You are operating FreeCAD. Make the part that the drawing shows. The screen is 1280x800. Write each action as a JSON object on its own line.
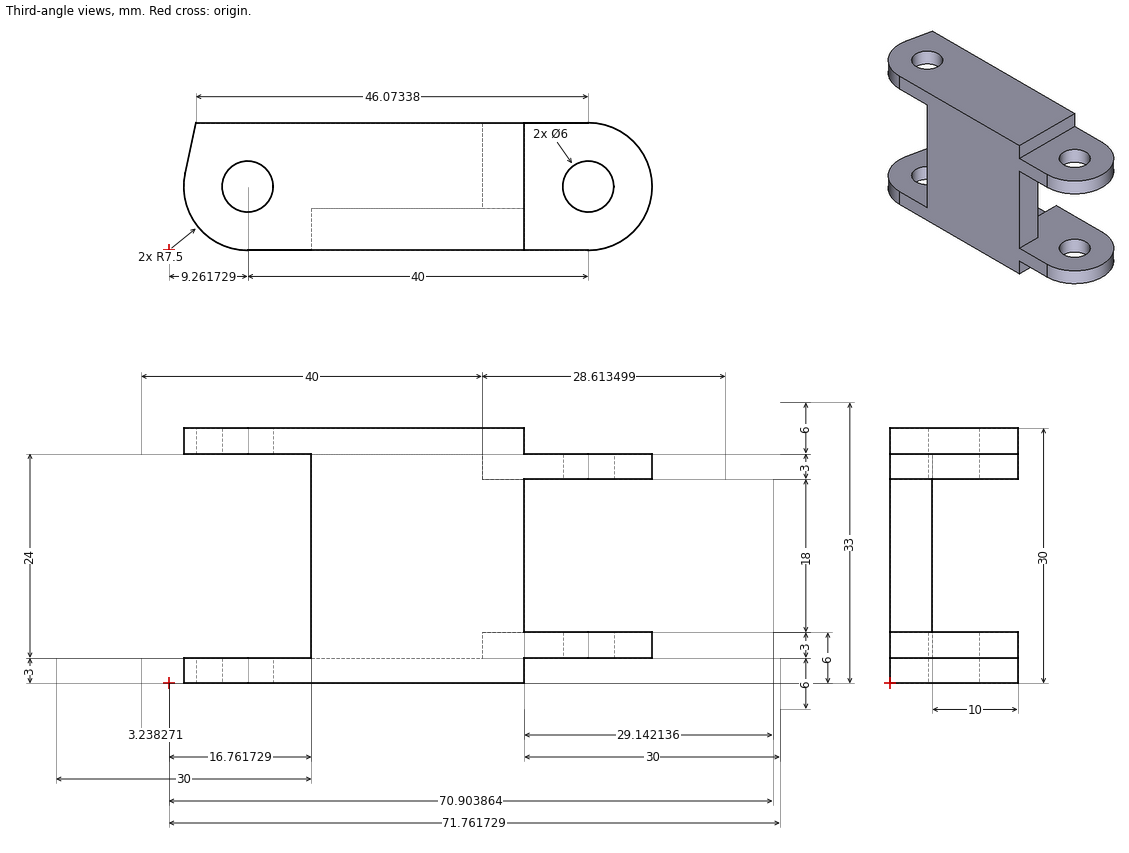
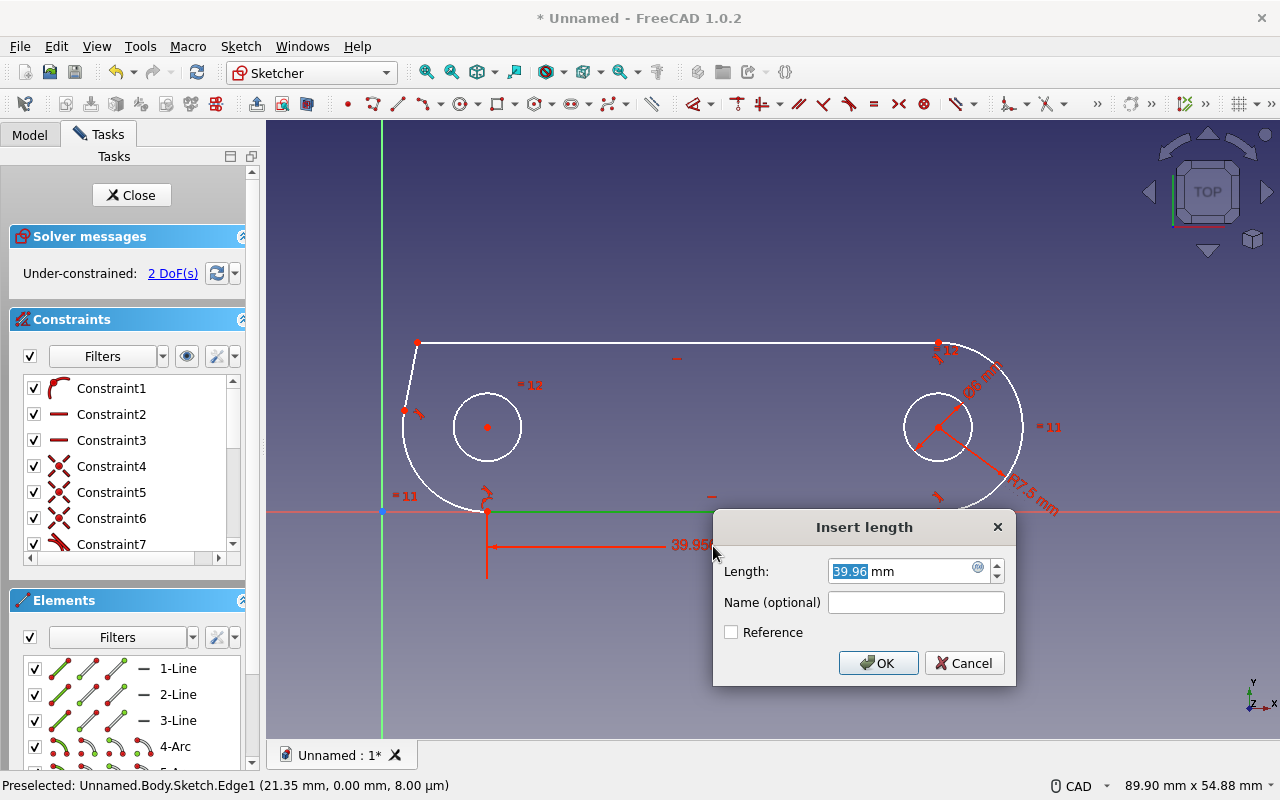
{"action": "type", "text": "40"}
{"action": "key", "text": "Return"}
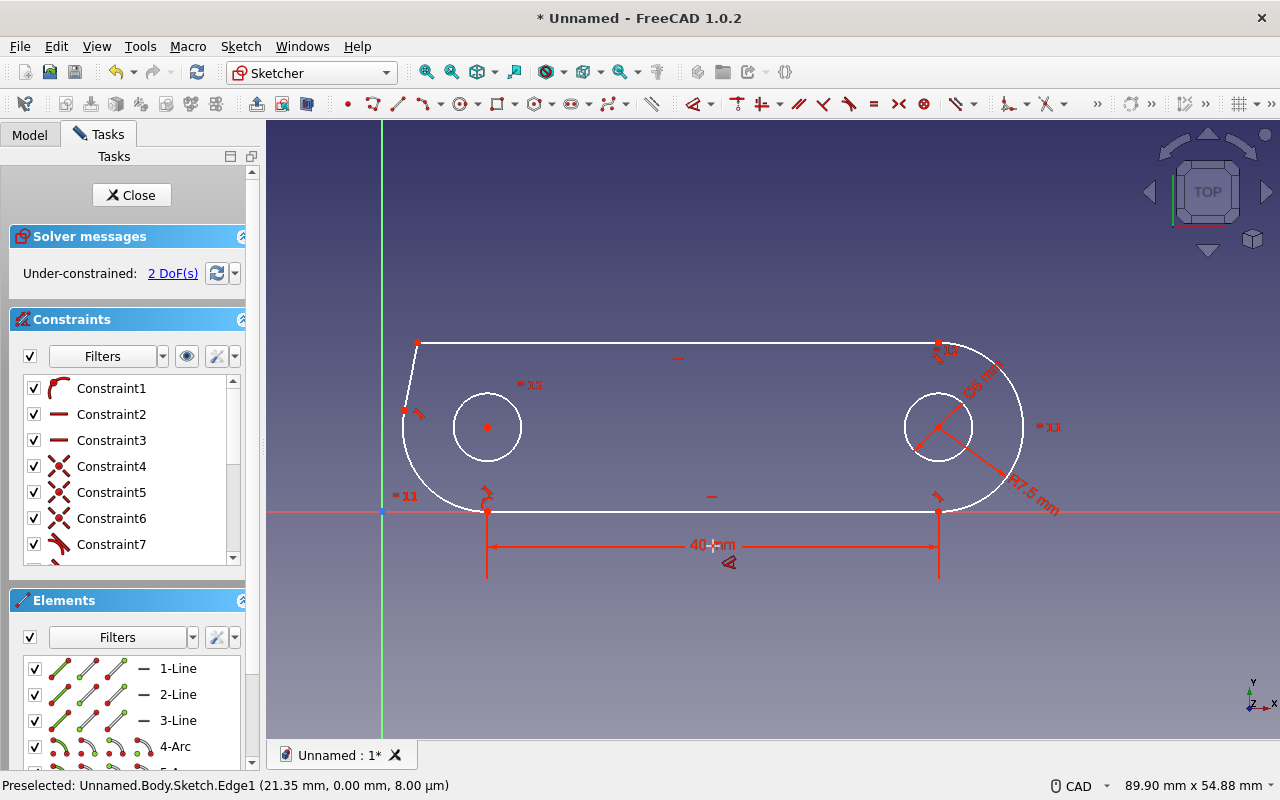
{"action": "left_click", "coordinate": [782, 343]}
{"action": "left_click", "coordinate": [678, 309]}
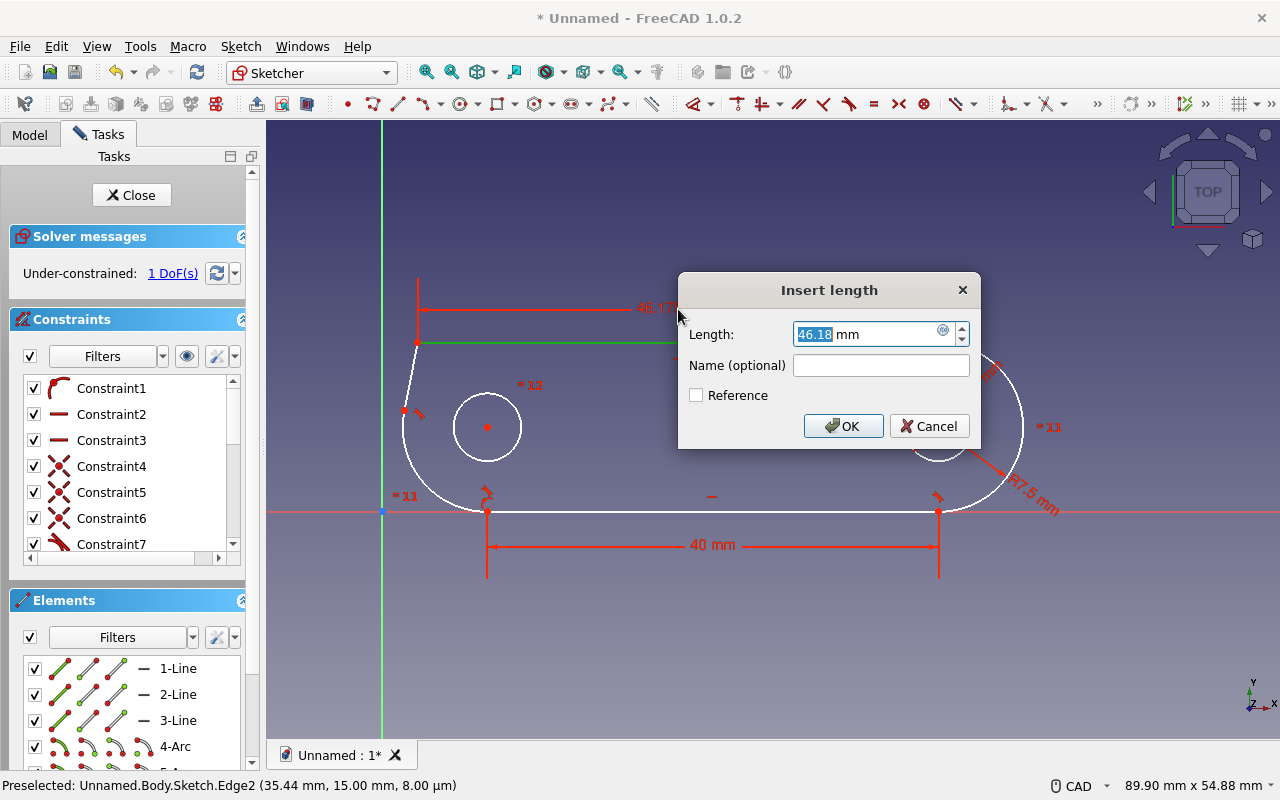
{"action": "type", "text": "46.07338"}
{"action": "key", "text": "Return"}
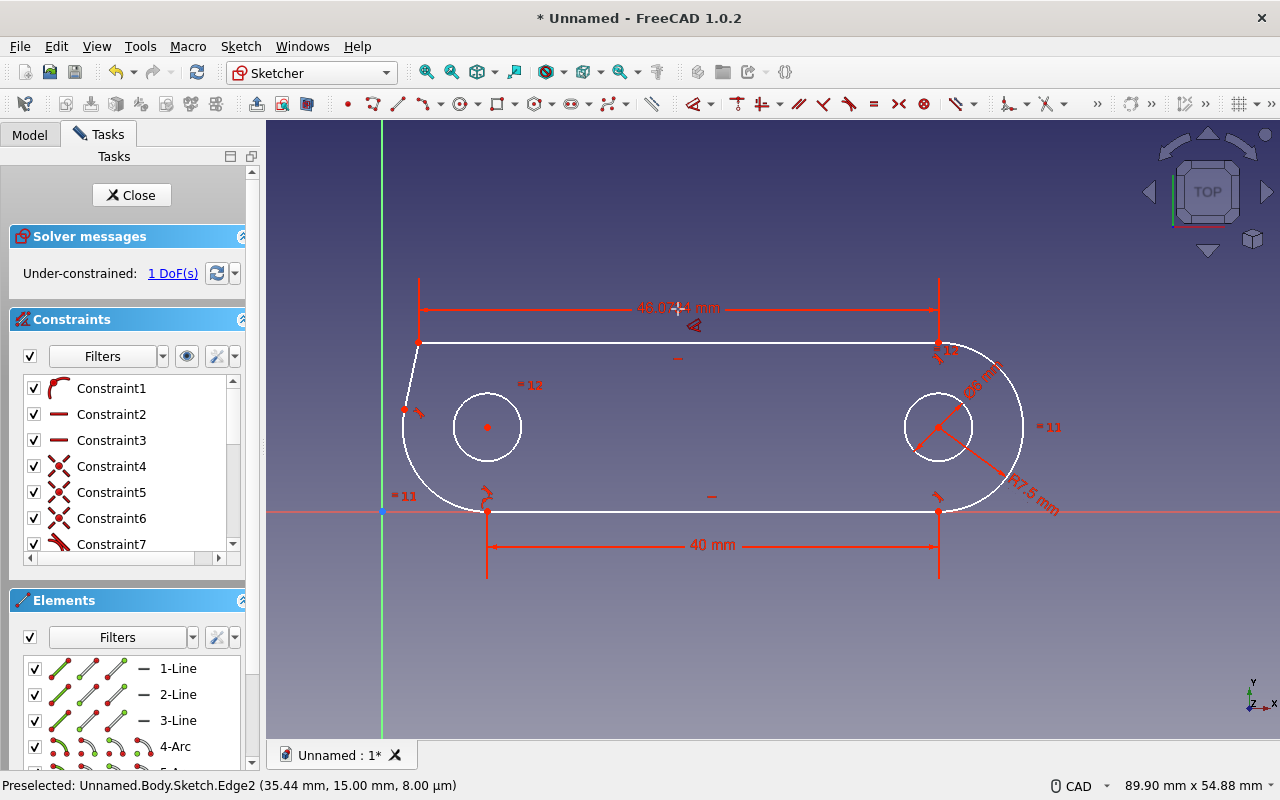
{"action": "left_click", "coordinate": [487, 427]}
{"action": "left_click", "coordinate": [435, 546]}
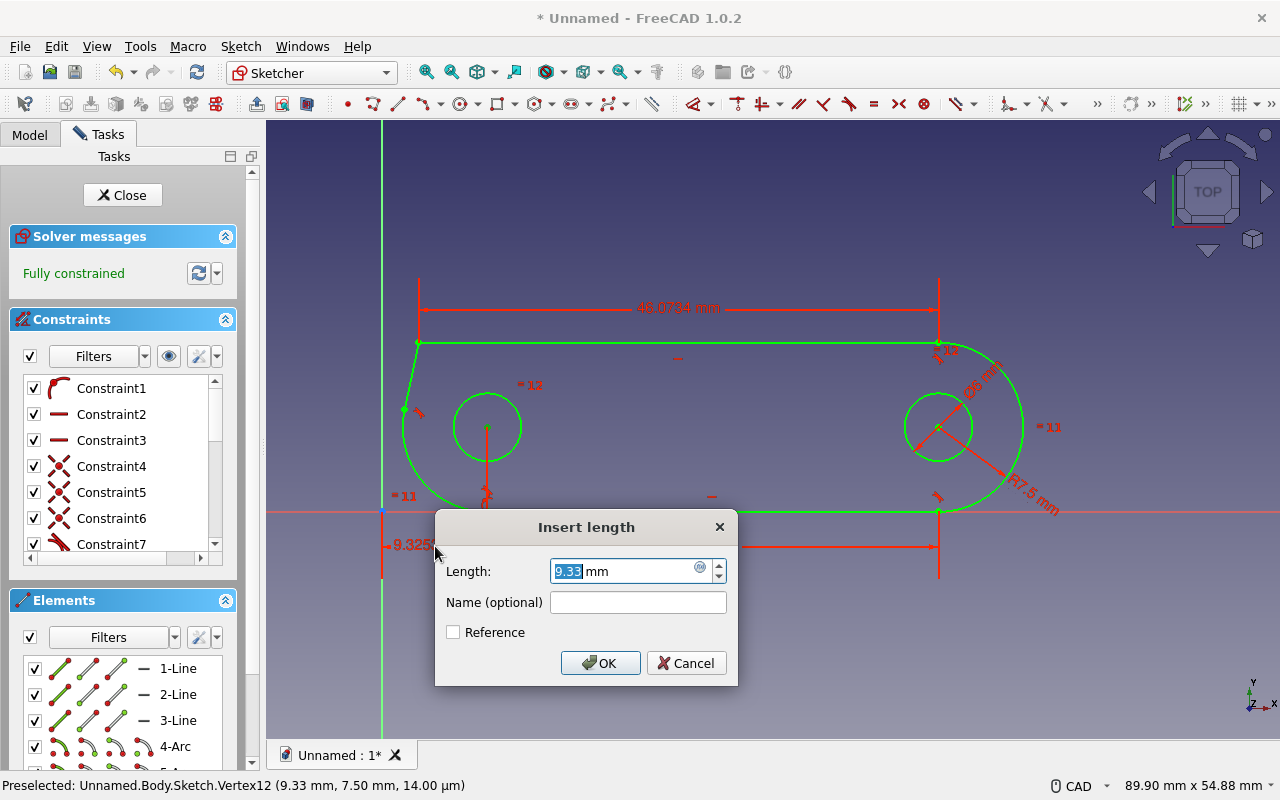
{"action": "type", "text": "9.261729"}
{"action": "key", "text": "Return"}
{"action": "key", "text": "Escape"}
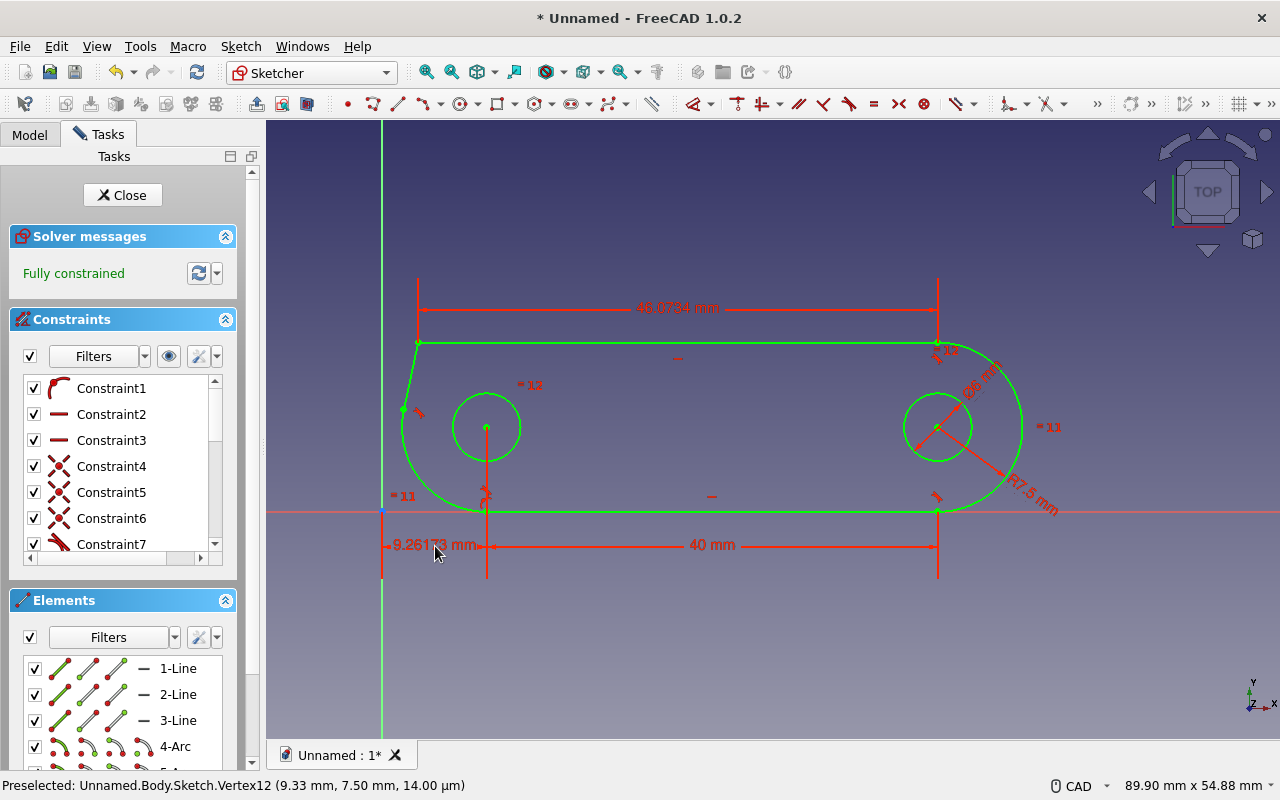
{"action": "left_click", "coordinate": [123, 195]}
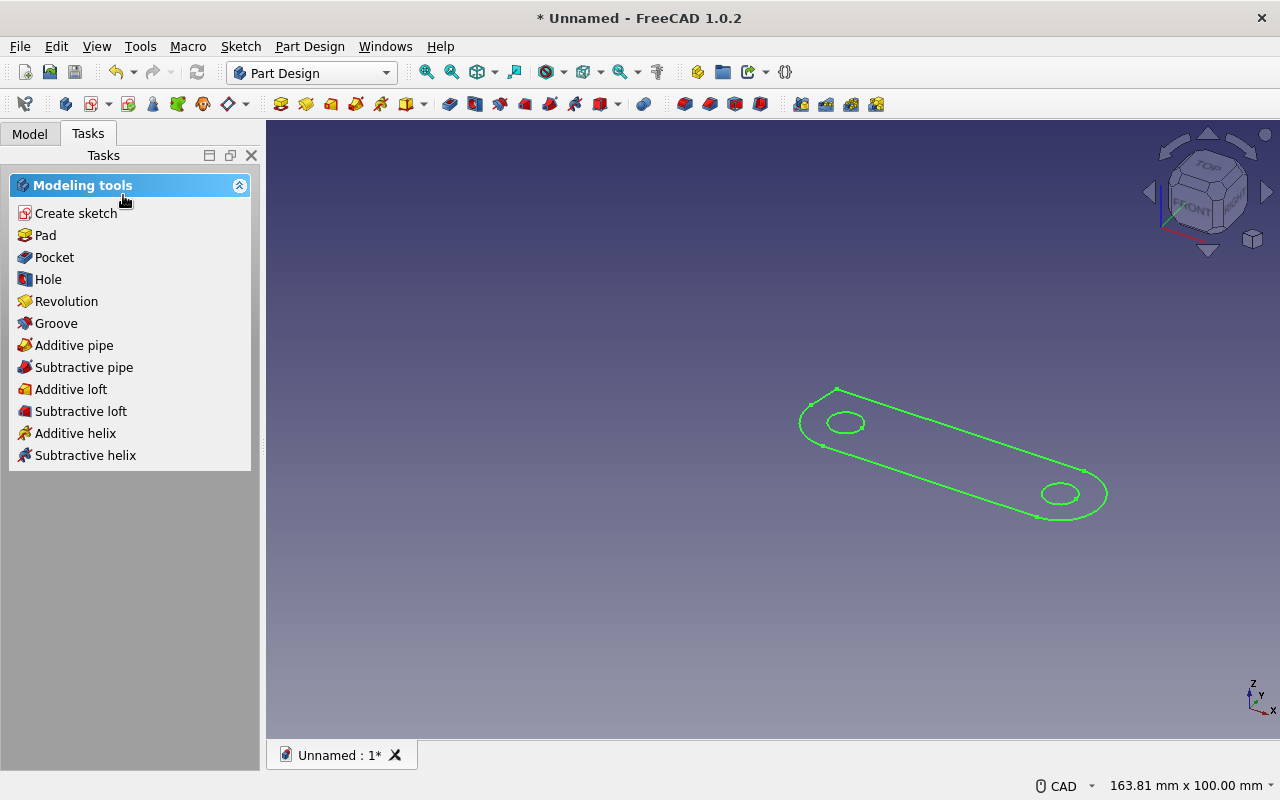
{"action": "left_click", "coordinate": [281, 104]}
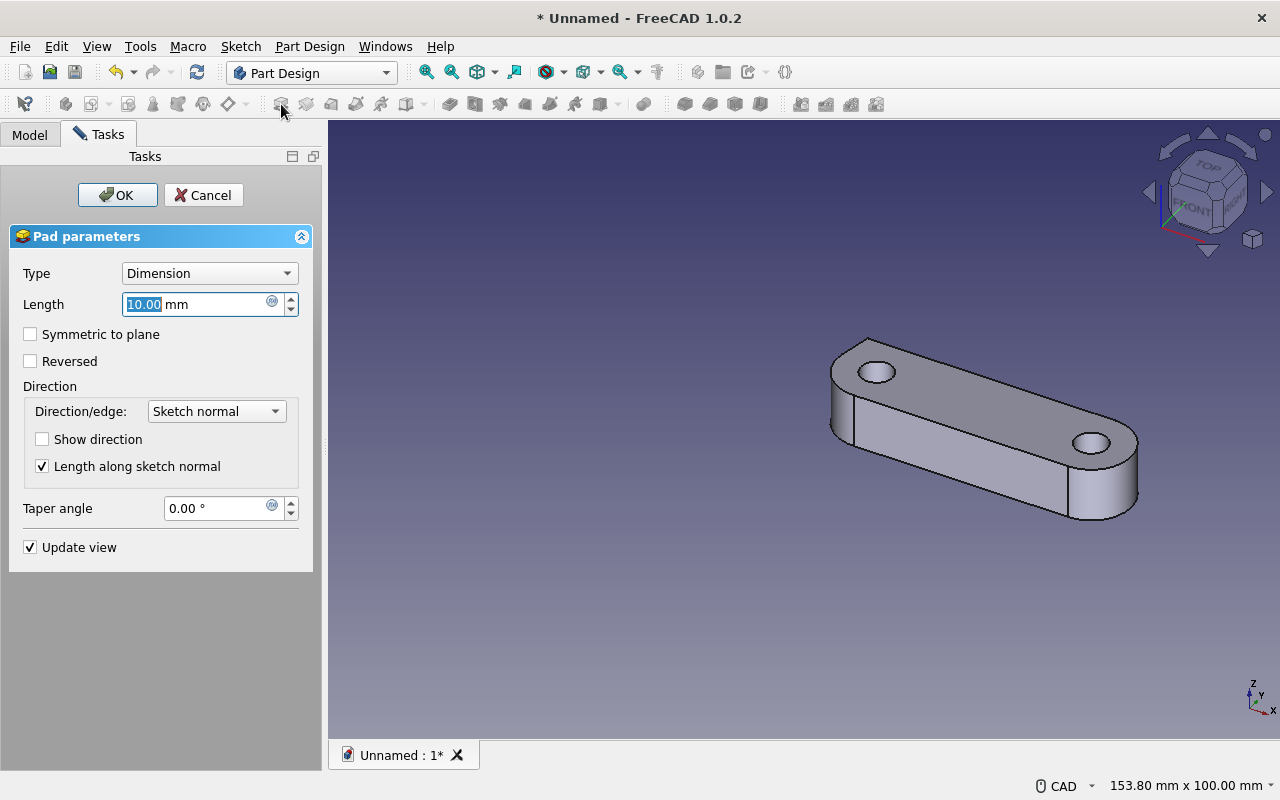
{"action": "type", "text": "30"}
{"action": "key", "text": "Tab"}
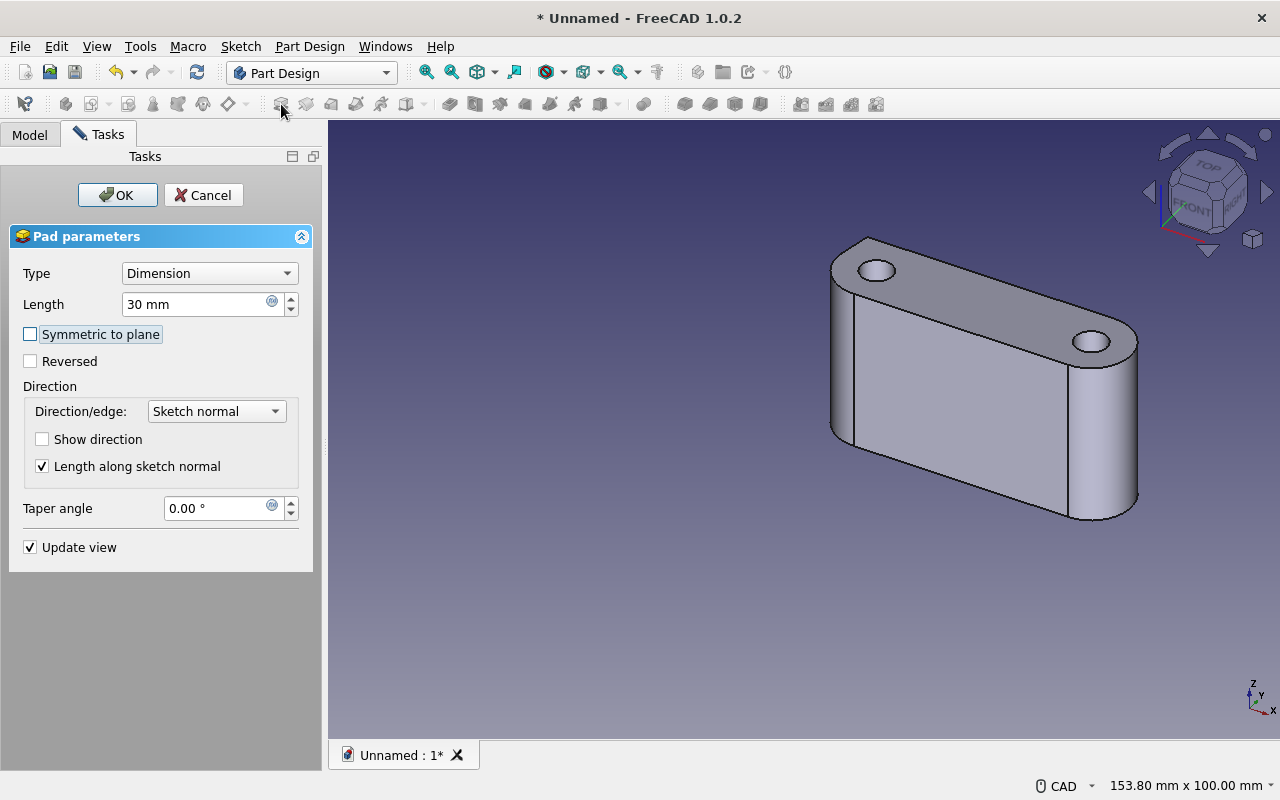
{"action": "left_click", "coordinate": [118, 195]}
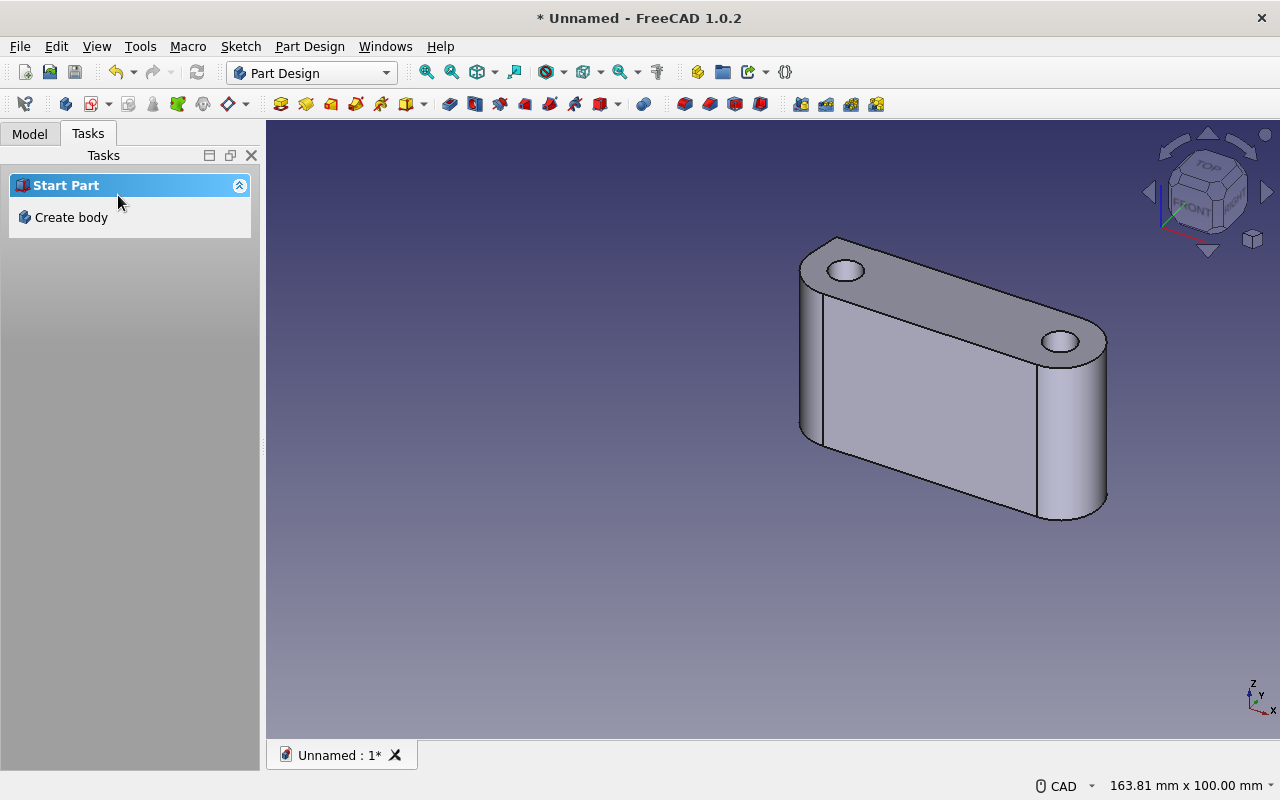
{"action": "key", "text": "4"}